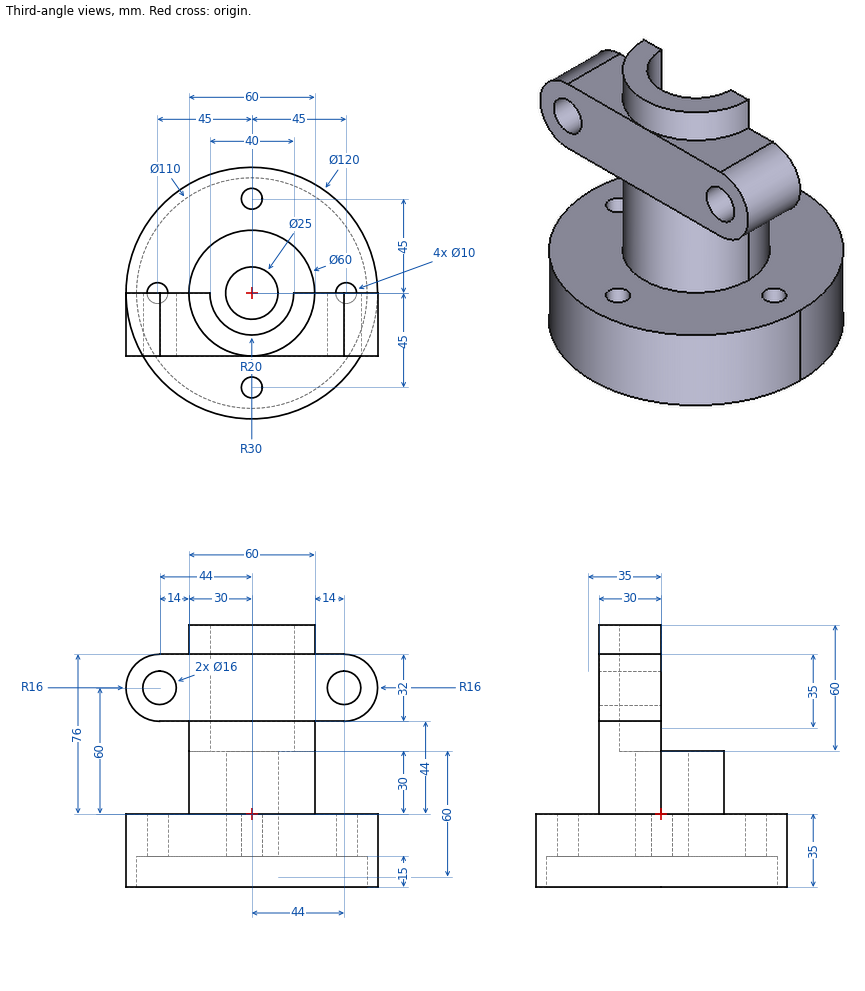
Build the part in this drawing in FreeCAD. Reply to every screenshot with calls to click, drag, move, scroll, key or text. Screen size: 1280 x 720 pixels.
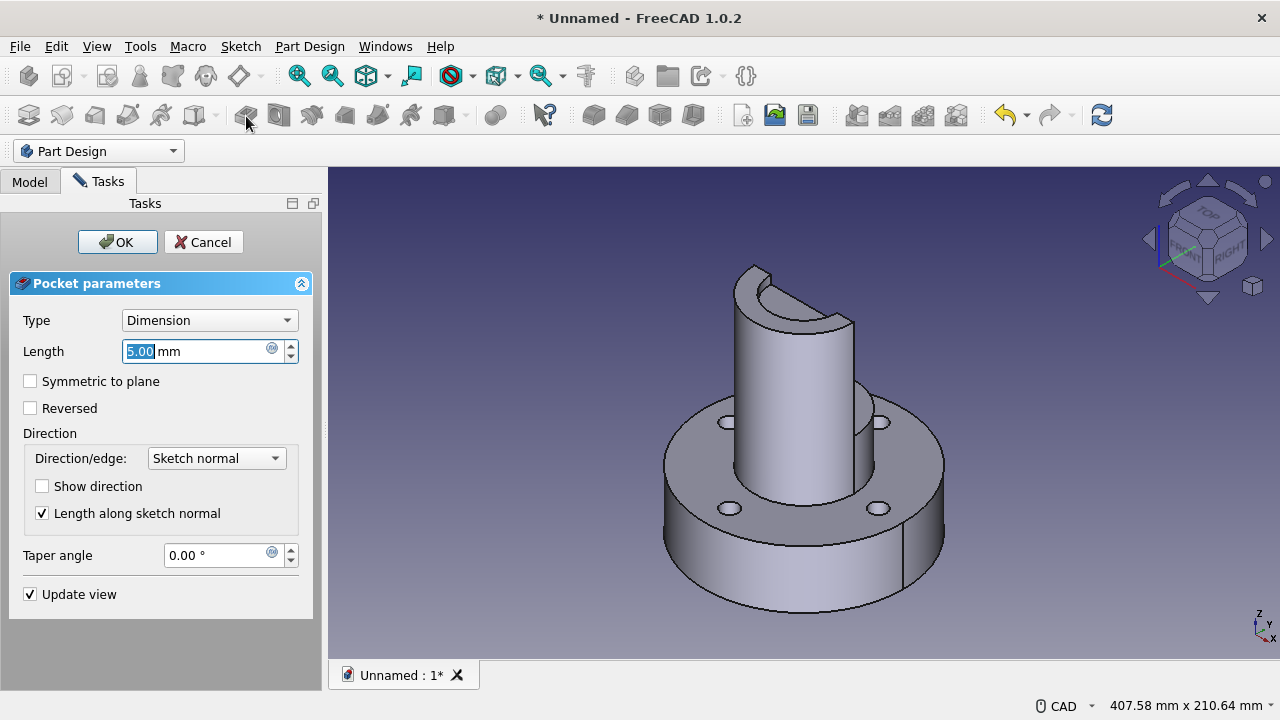
text(60)
key(Tab)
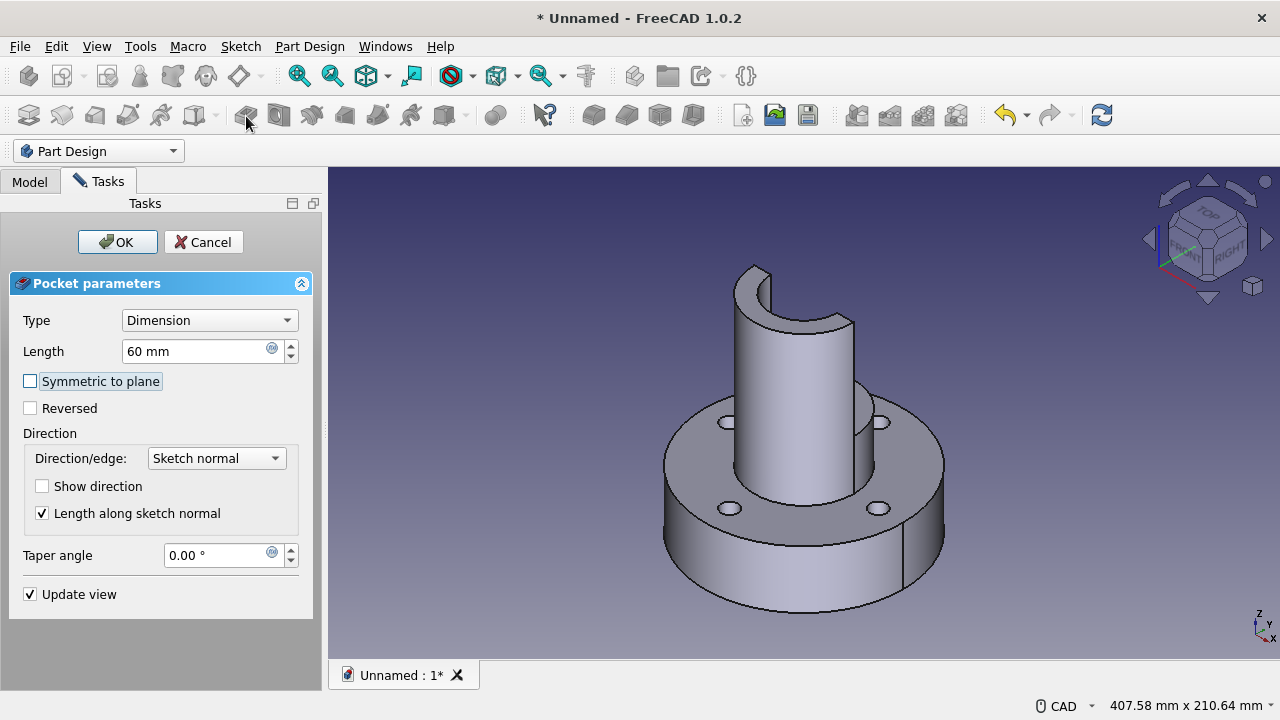
click(118, 242)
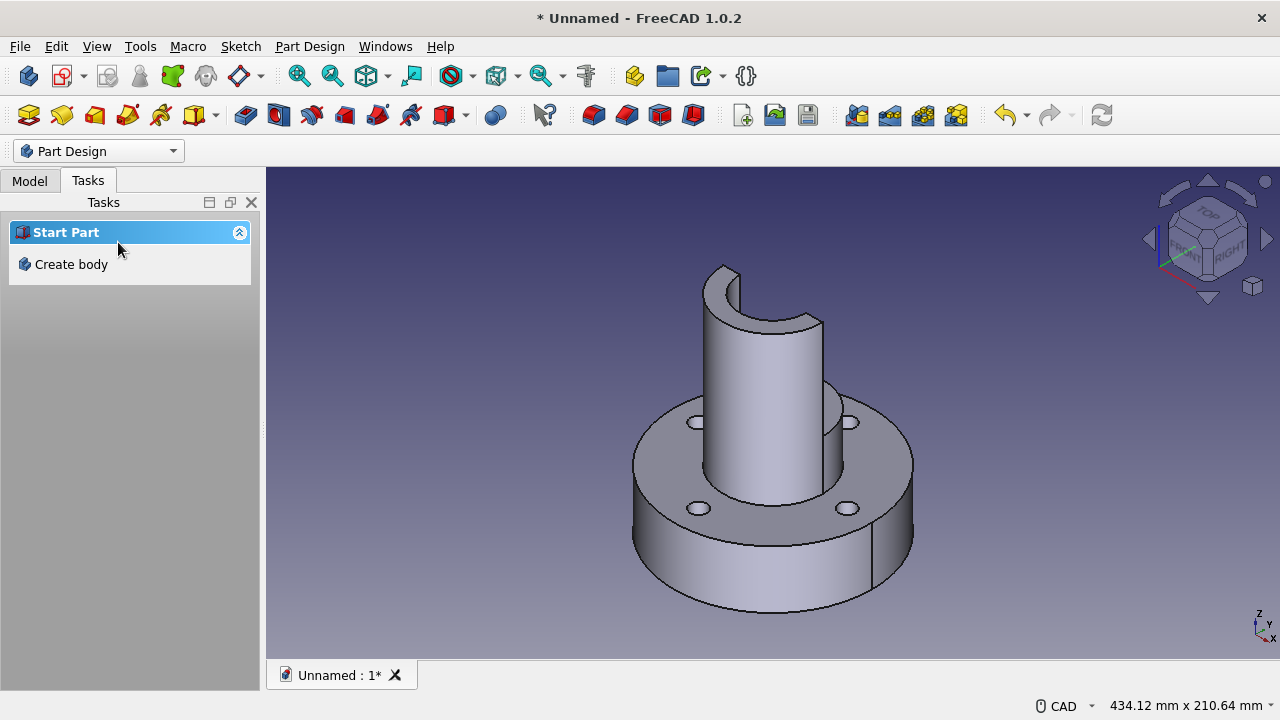
key(2)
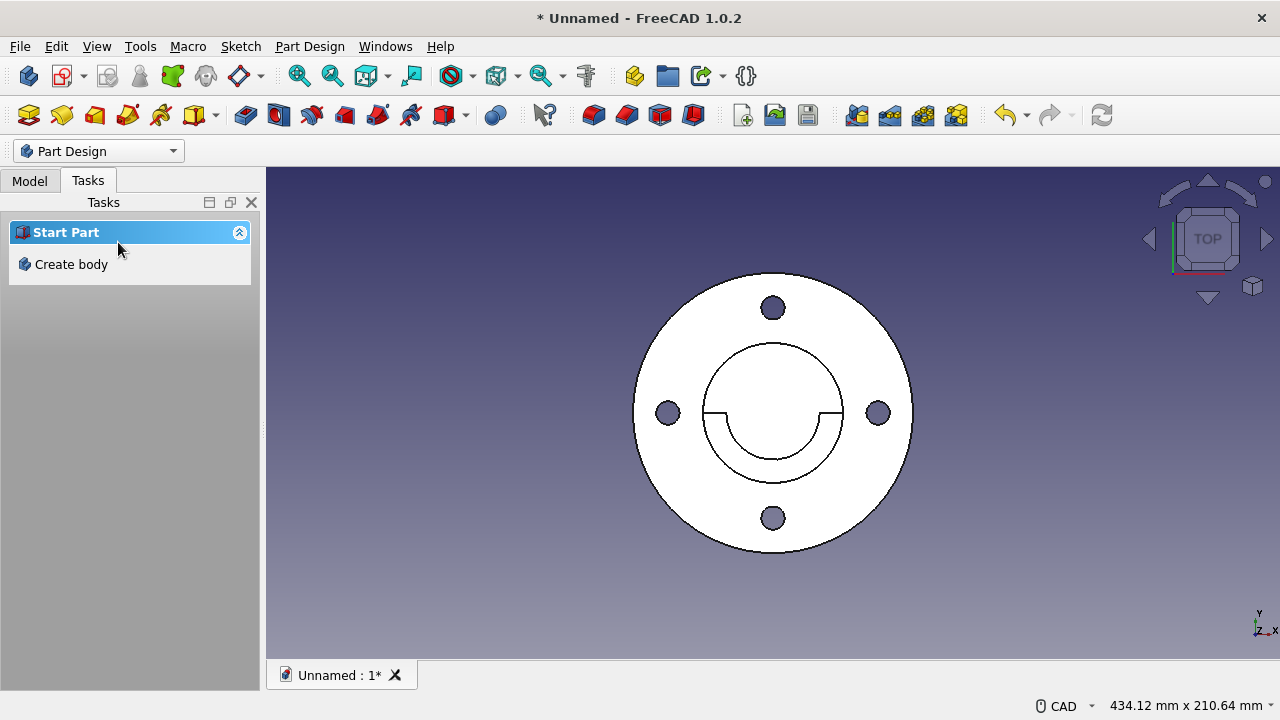
click(773, 400)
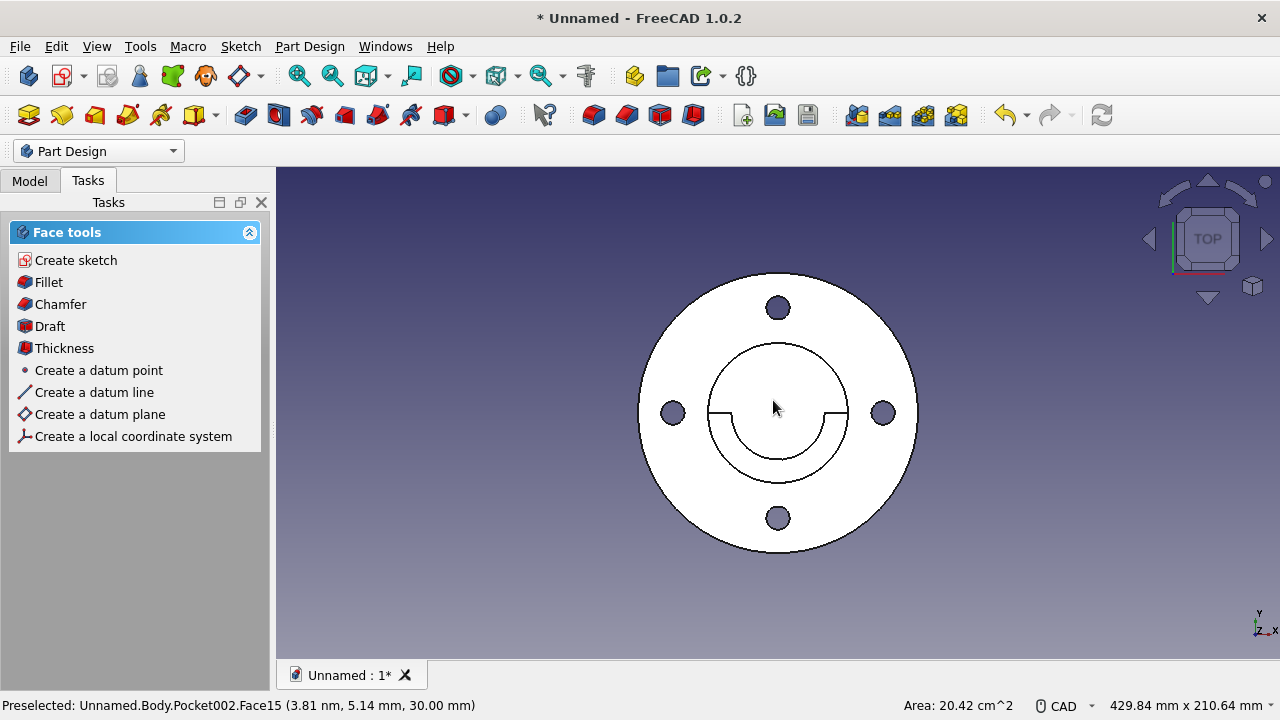
click(62, 76)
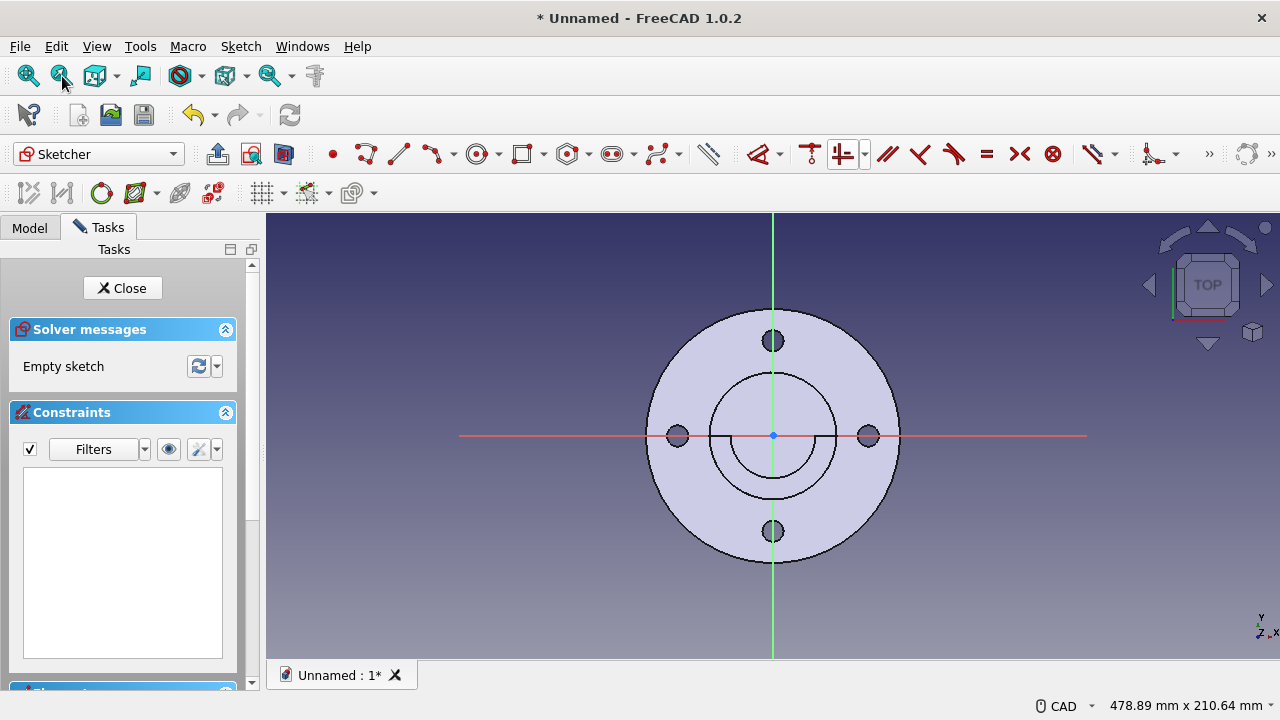
scroll(790, 436, up, 8)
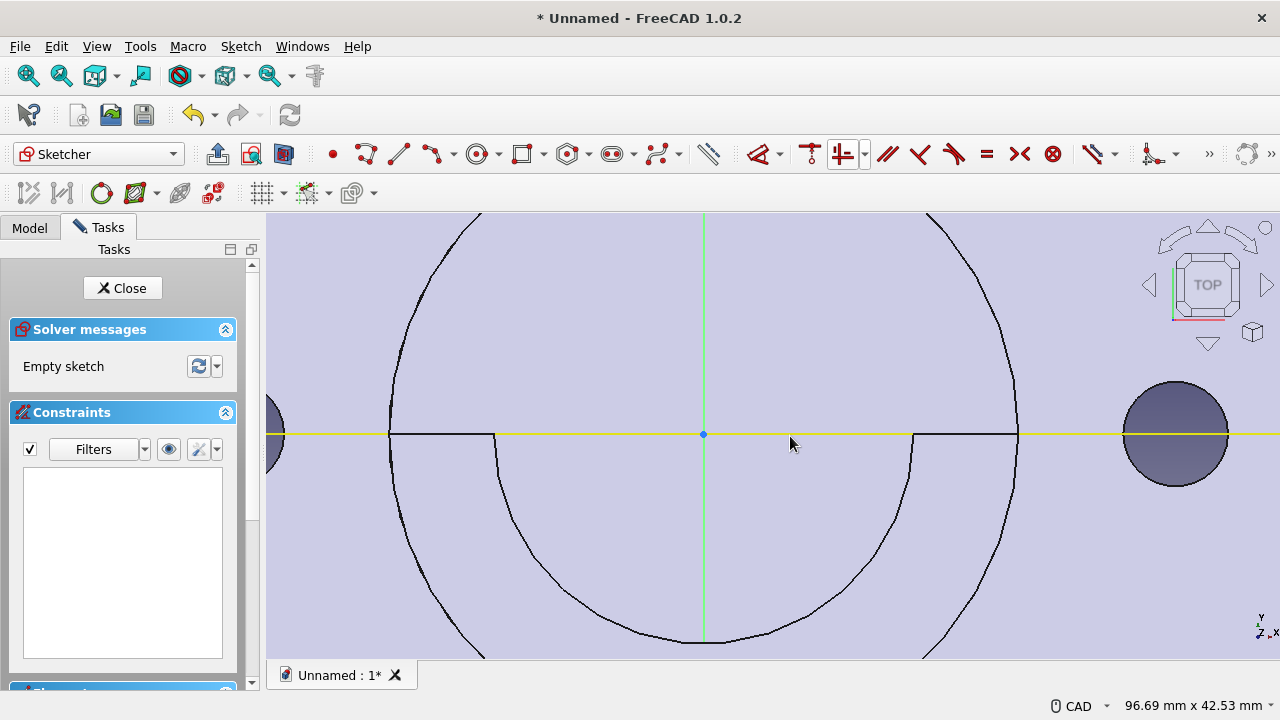
click(476, 154)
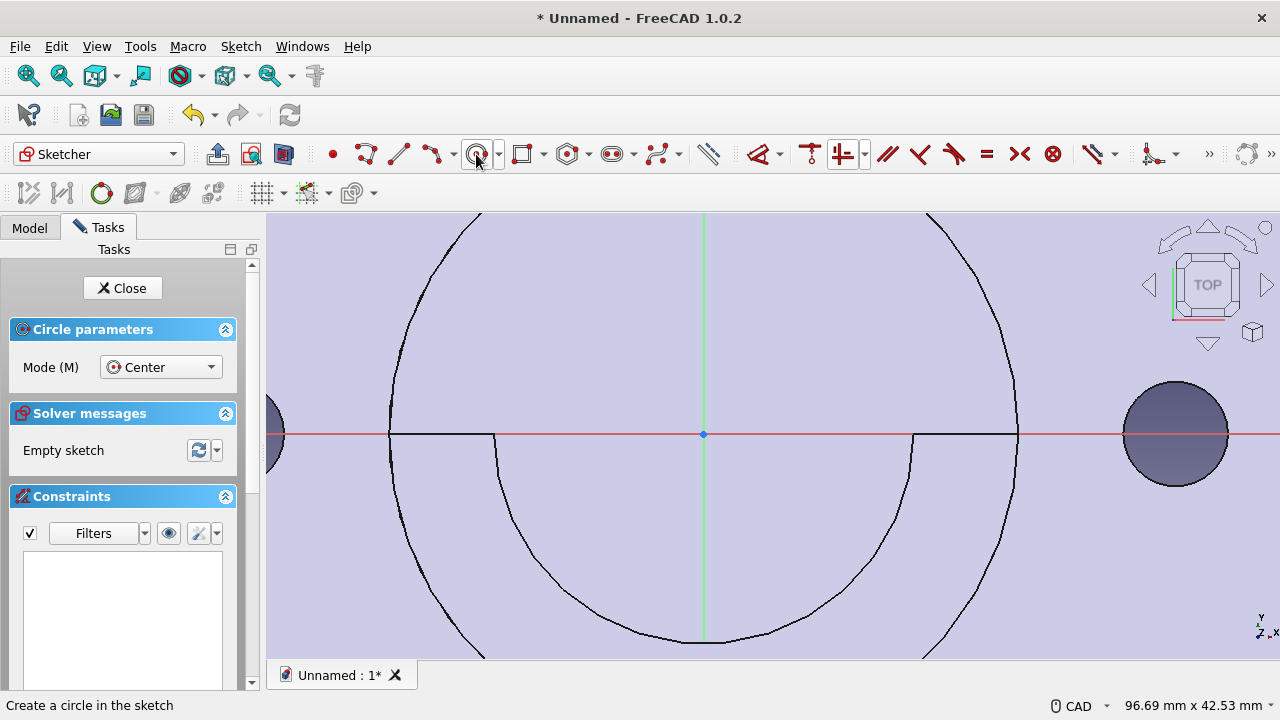
click(704, 434)
move(796, 341)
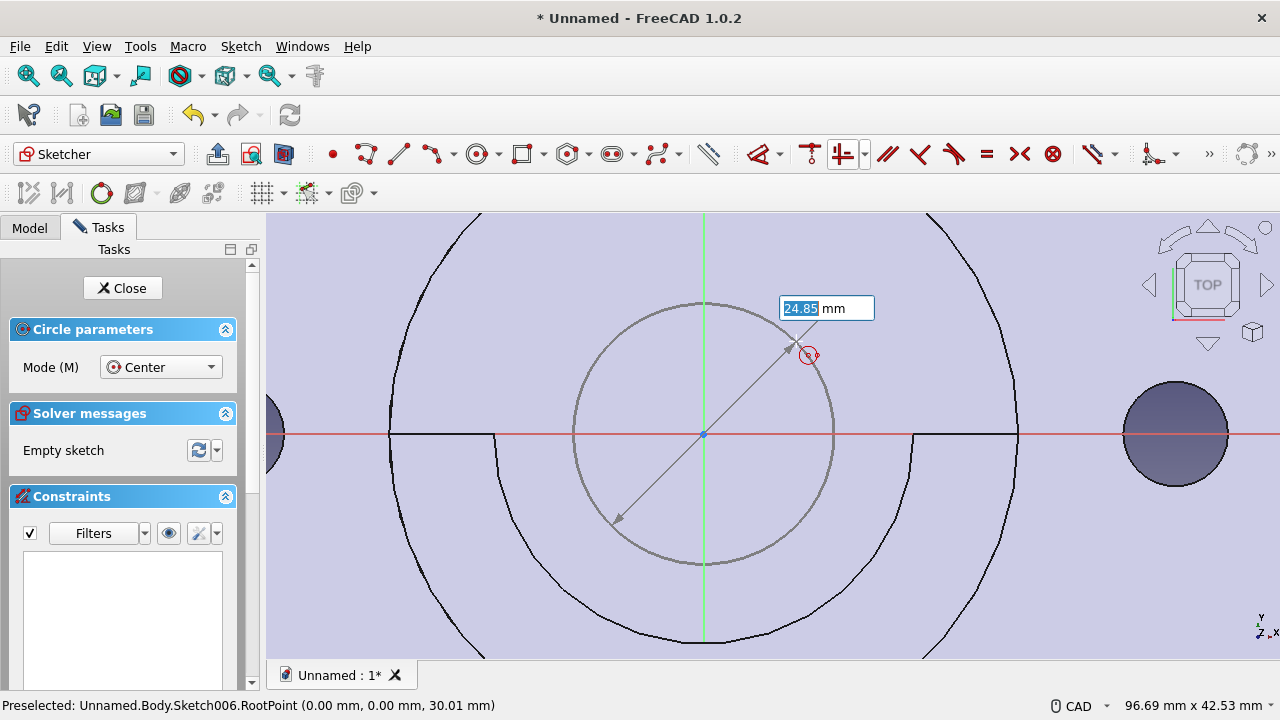
text(25)
key(Return)
key(Escape)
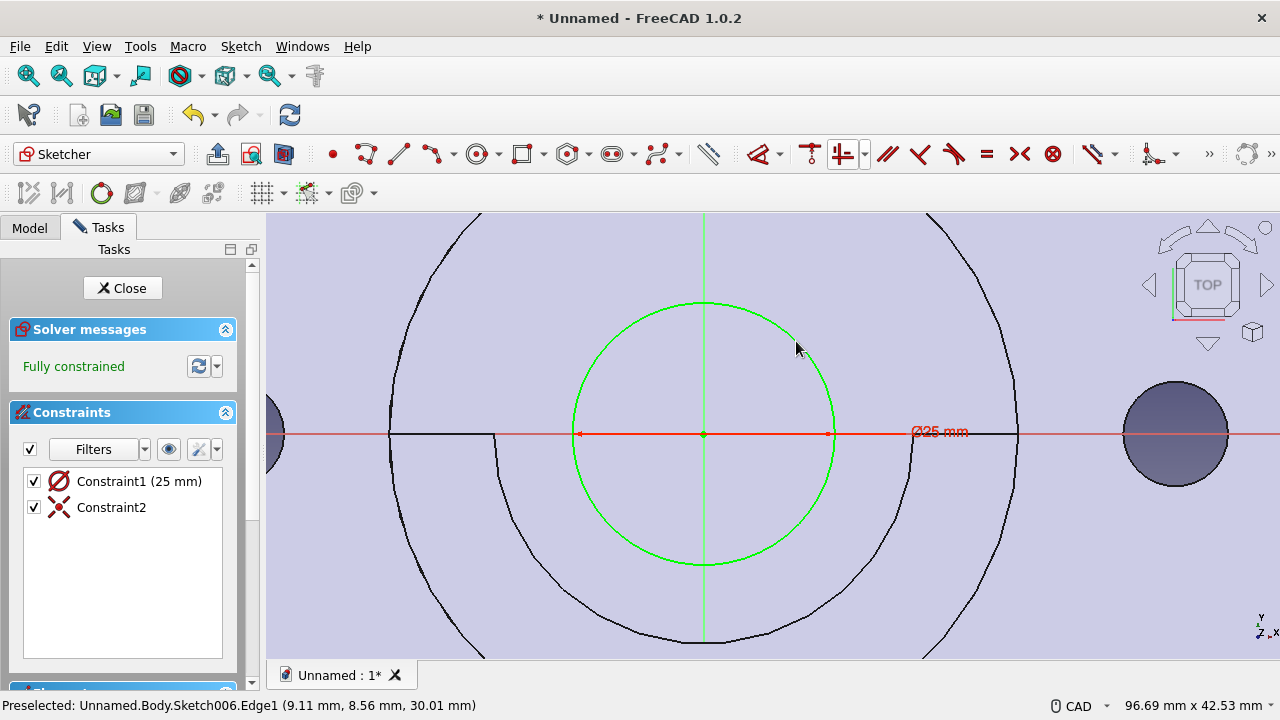
click(123, 288)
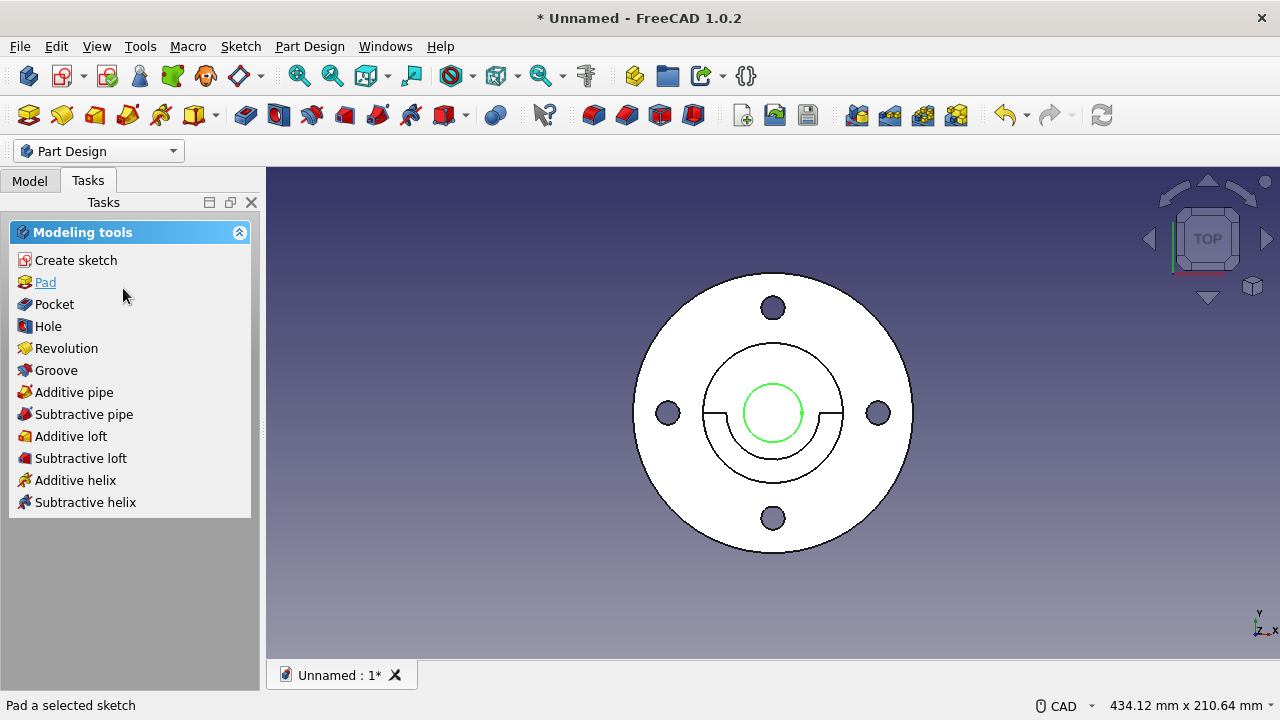
click(246, 116)